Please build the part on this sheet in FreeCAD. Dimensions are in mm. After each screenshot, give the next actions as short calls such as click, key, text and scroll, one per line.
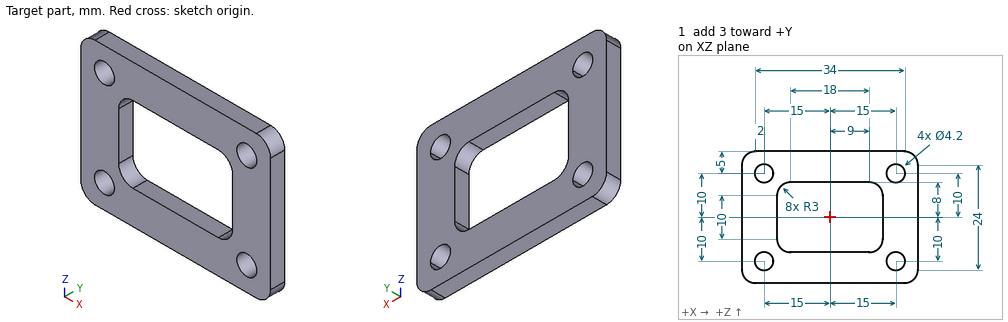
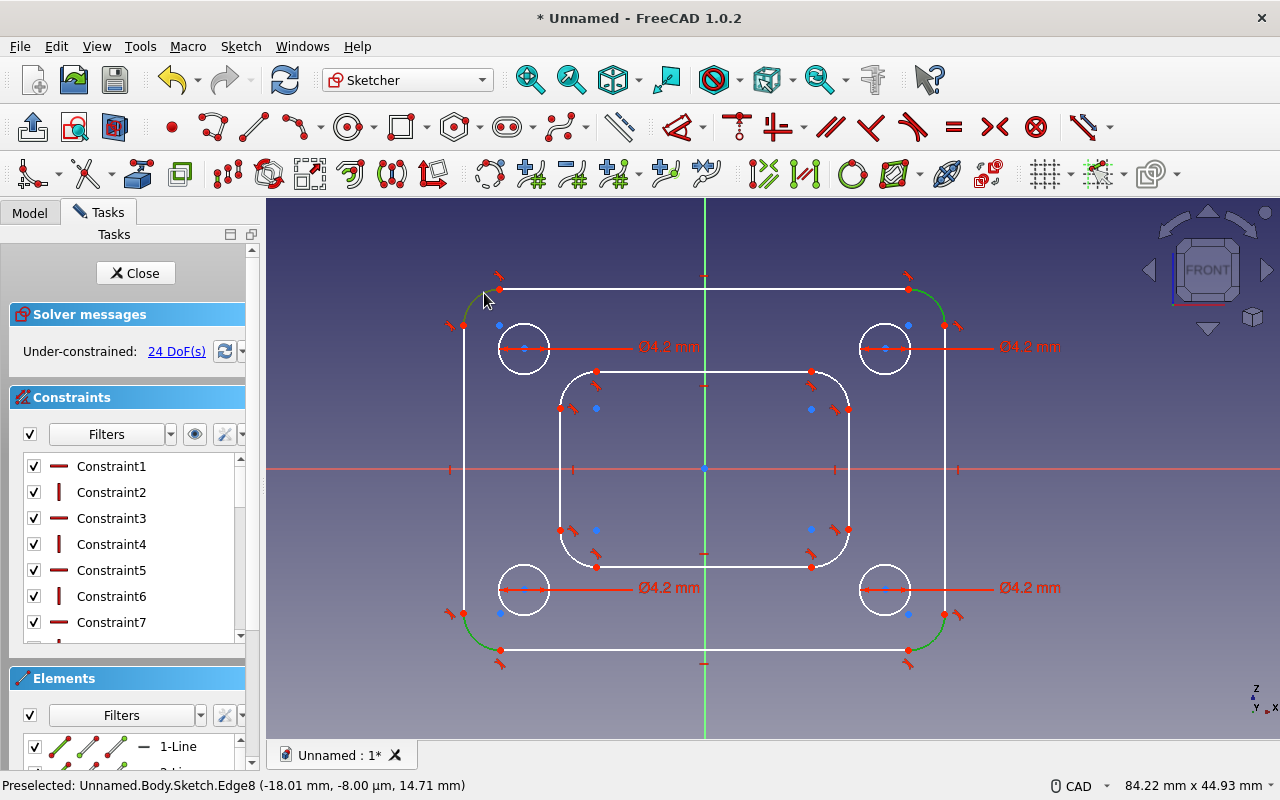
click(580, 376)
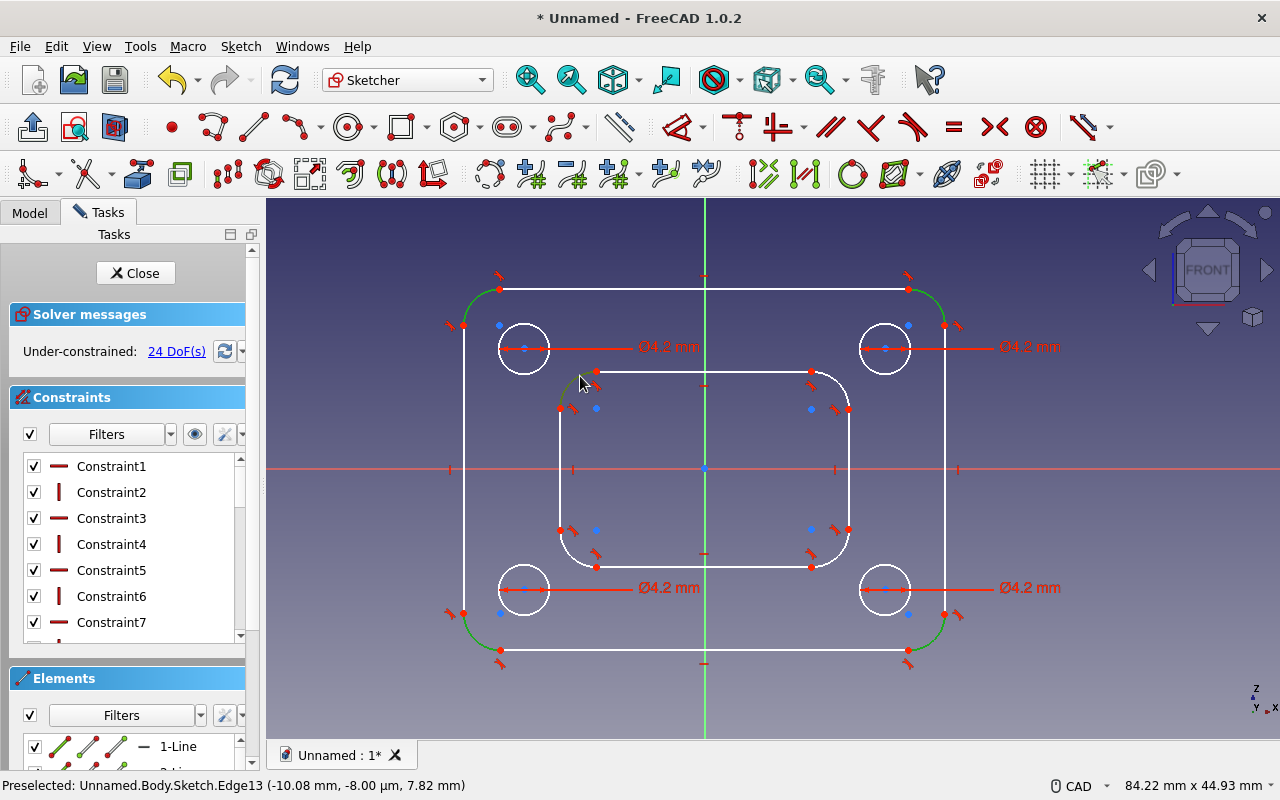
click(564, 547)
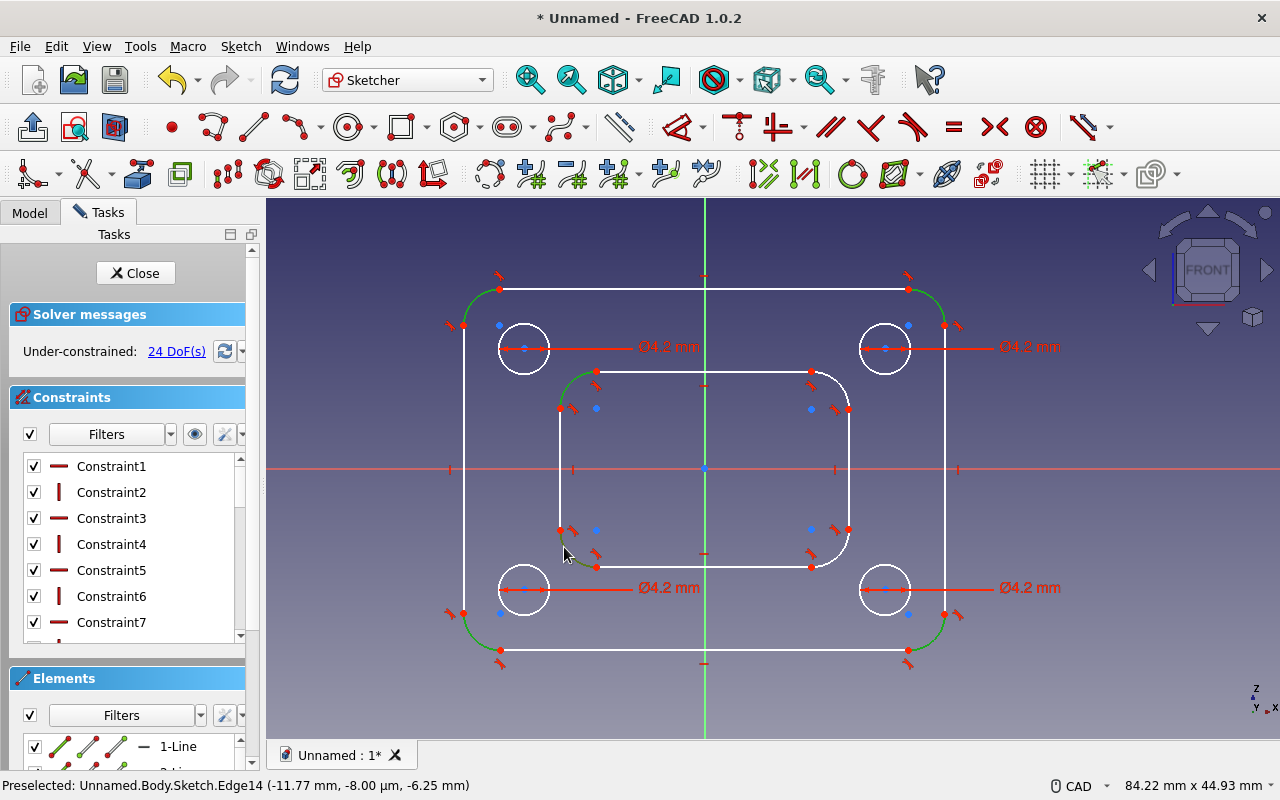
click(829, 563)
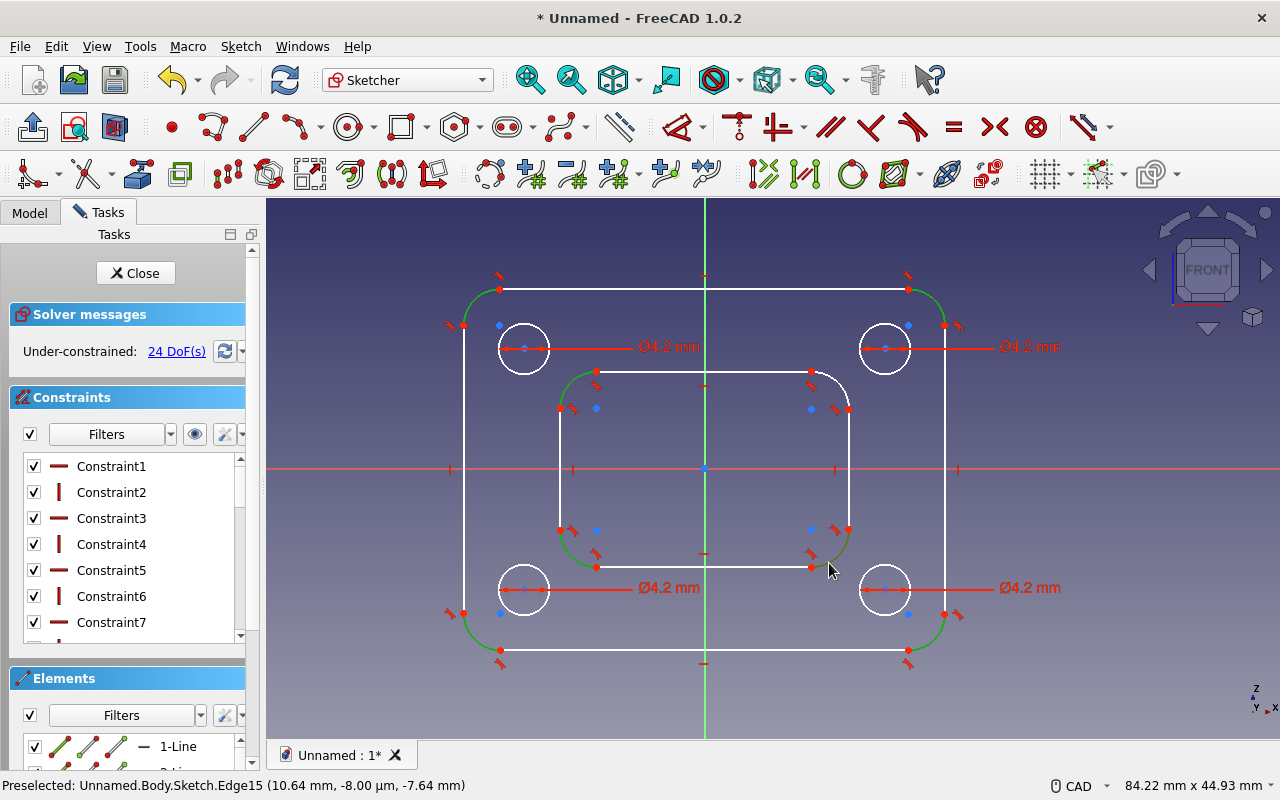
click(845, 392)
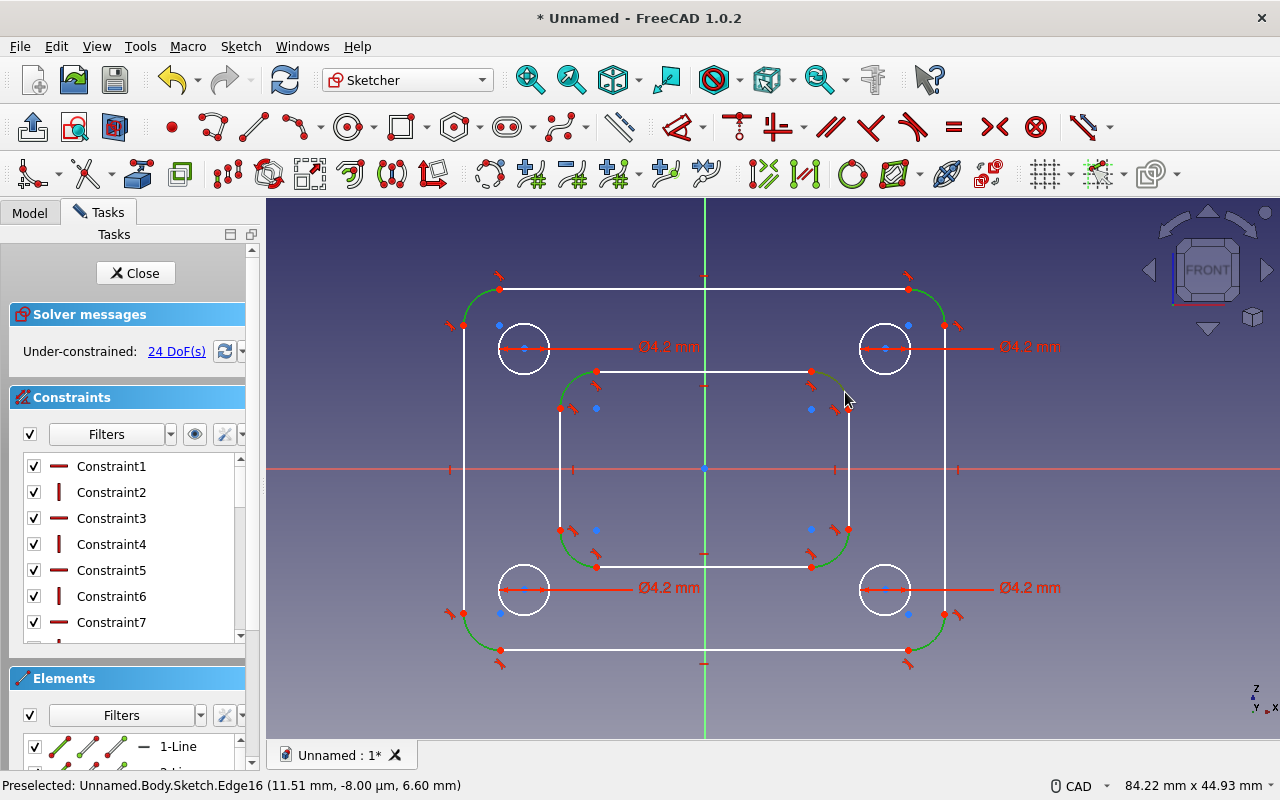
key(e)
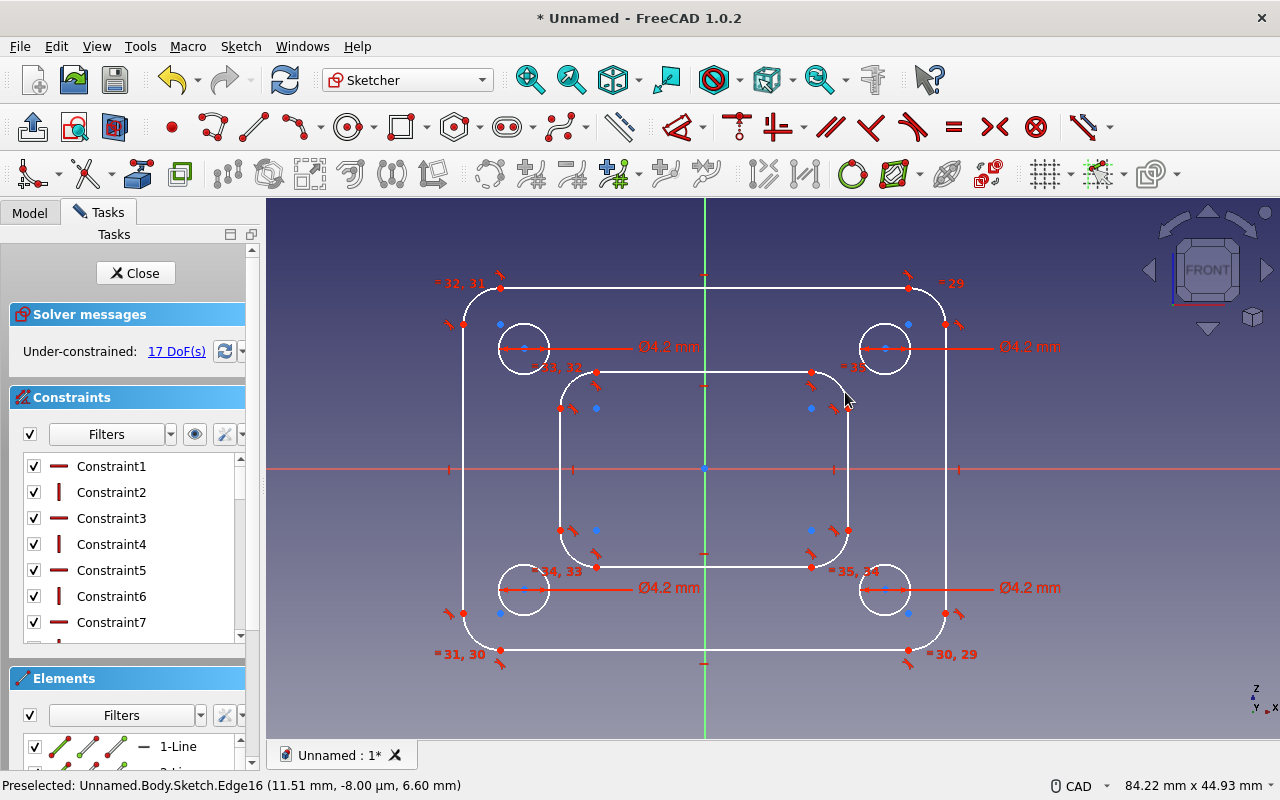
click(942, 308)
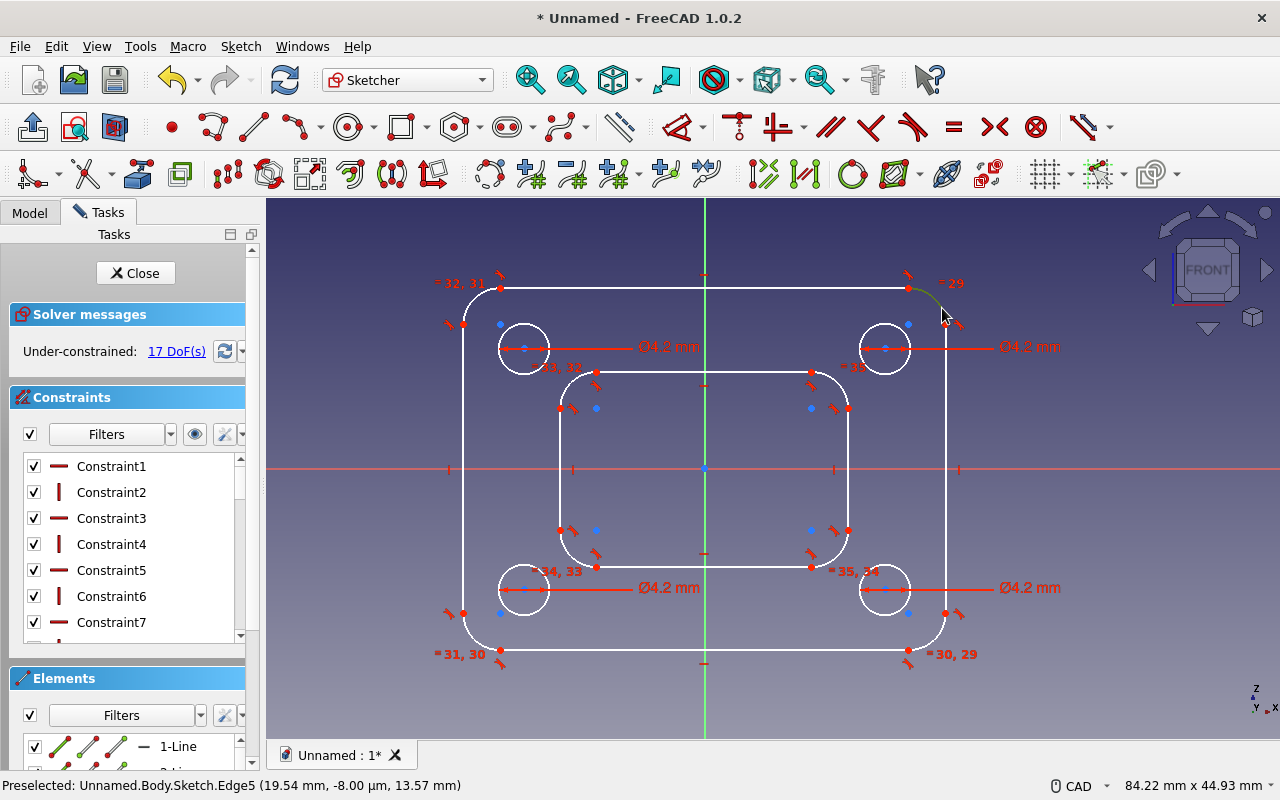
key(k)
key(r)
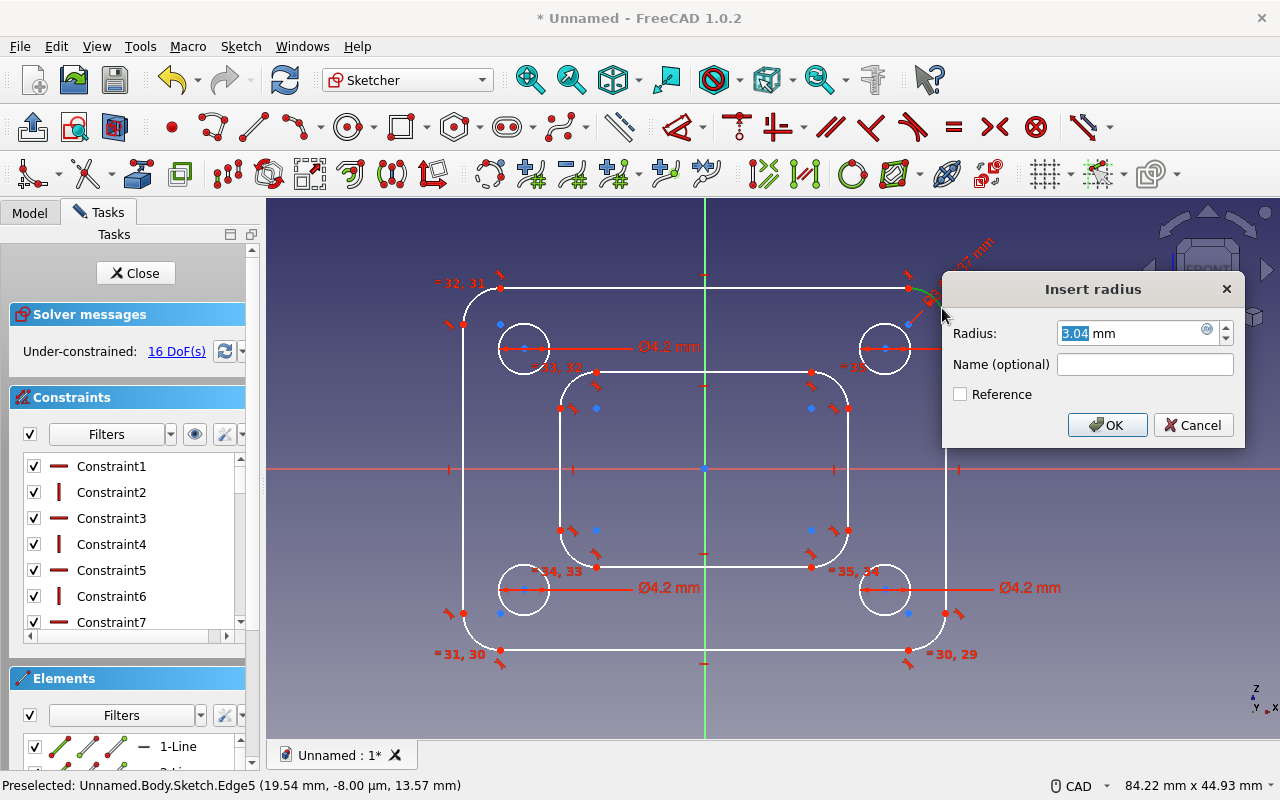
text(3)
key(Return)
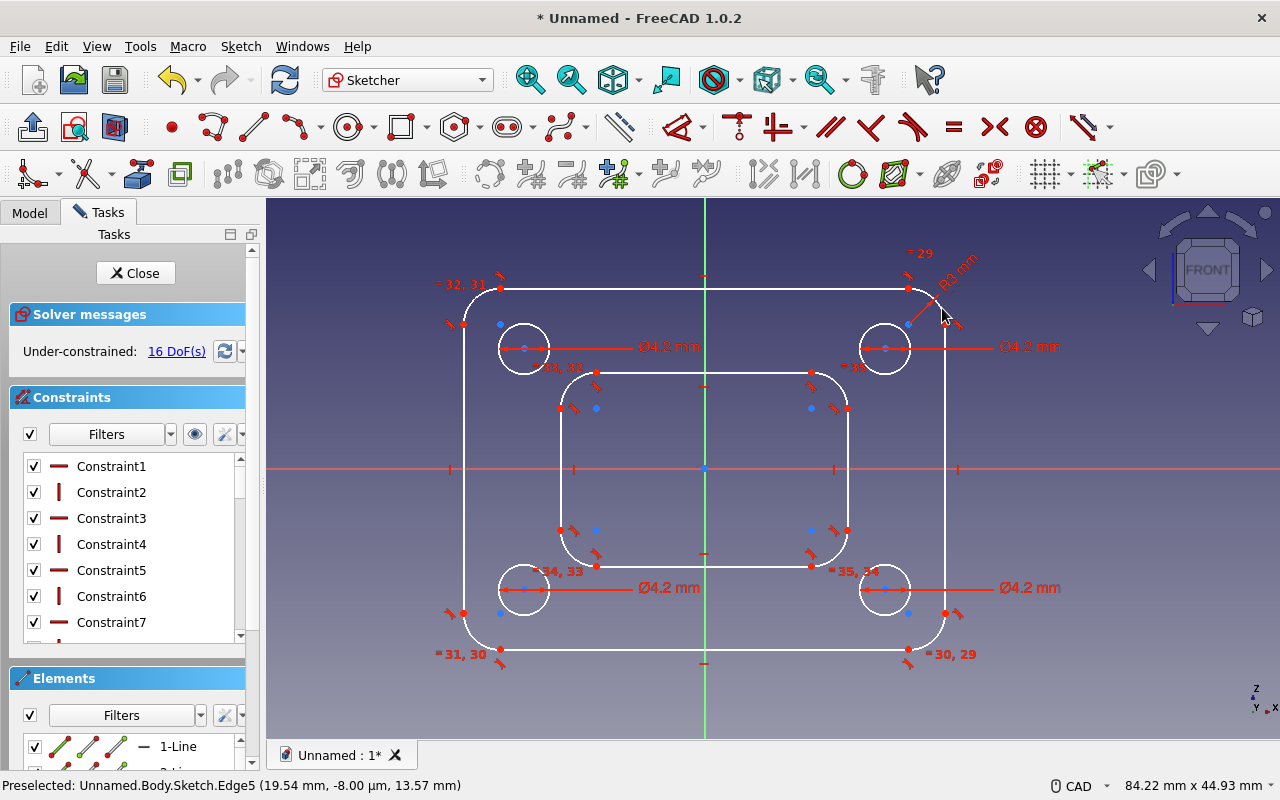
click(623, 289)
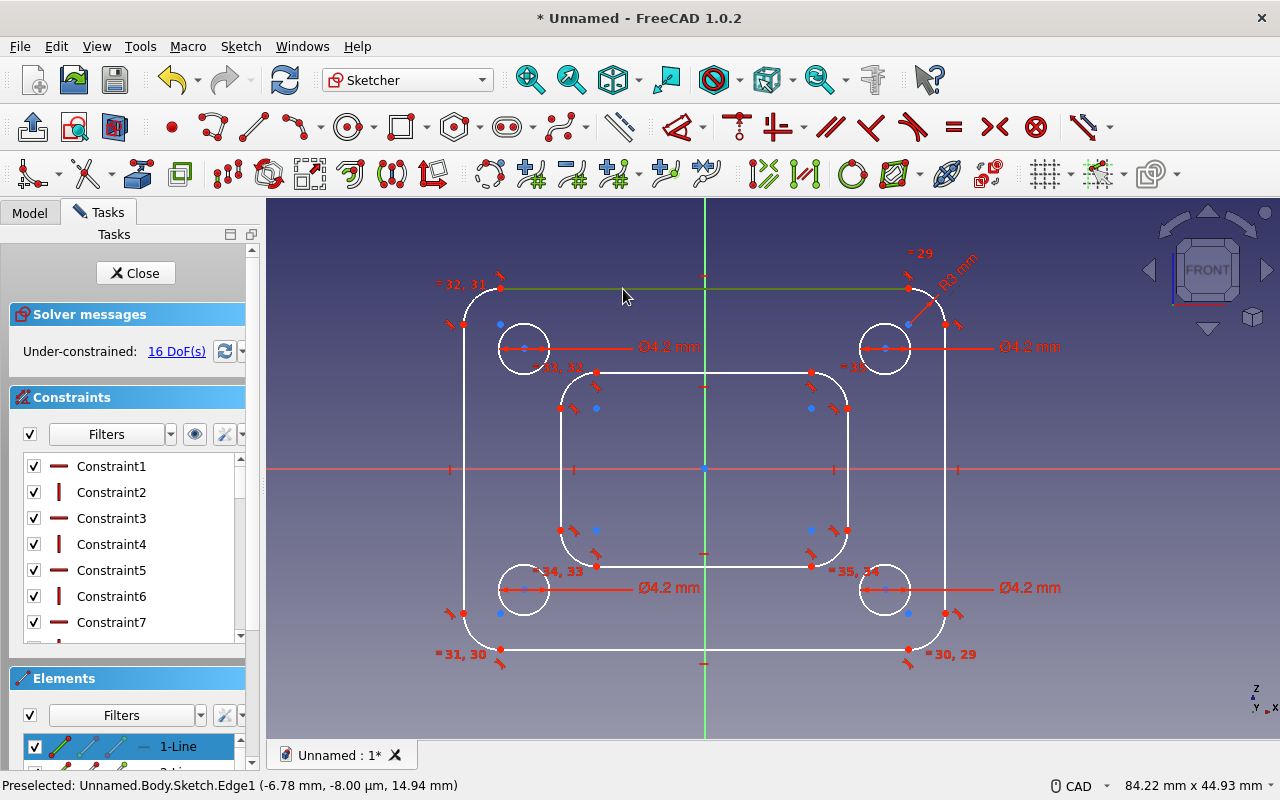
key(l)